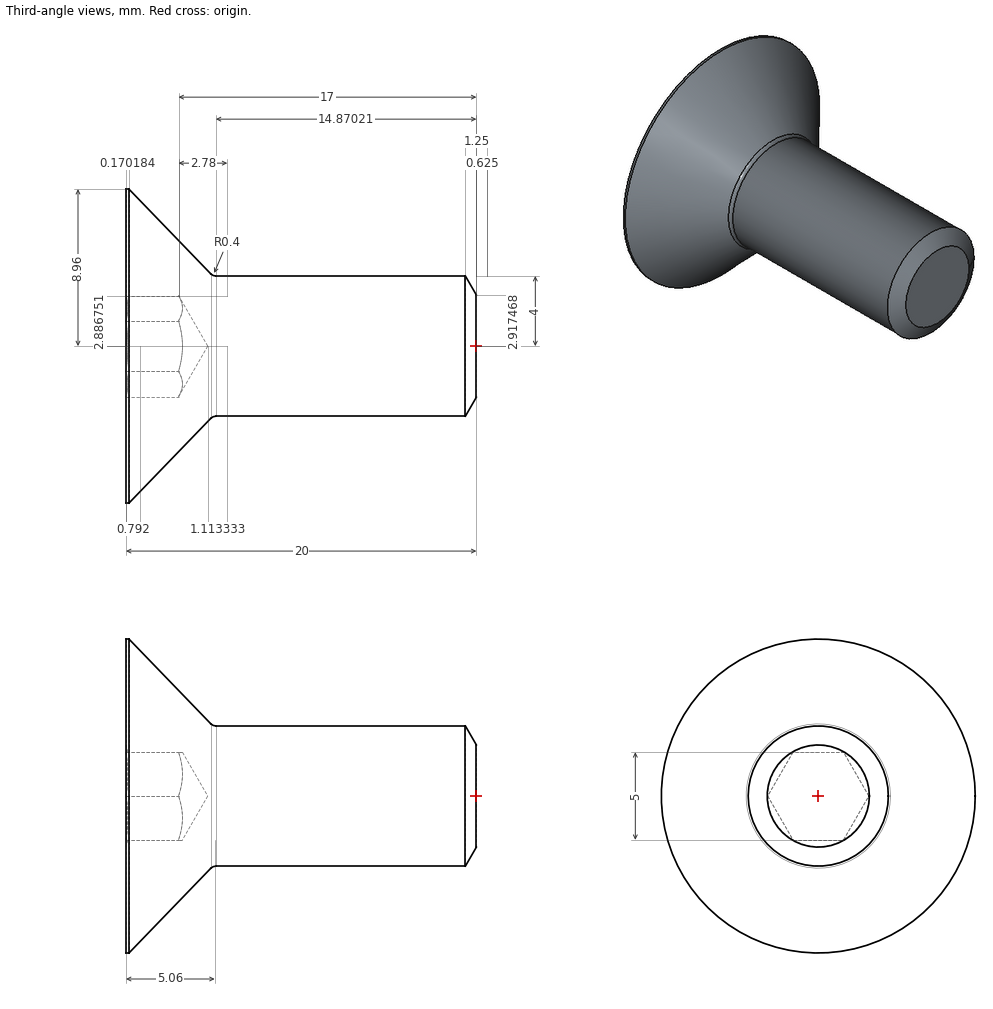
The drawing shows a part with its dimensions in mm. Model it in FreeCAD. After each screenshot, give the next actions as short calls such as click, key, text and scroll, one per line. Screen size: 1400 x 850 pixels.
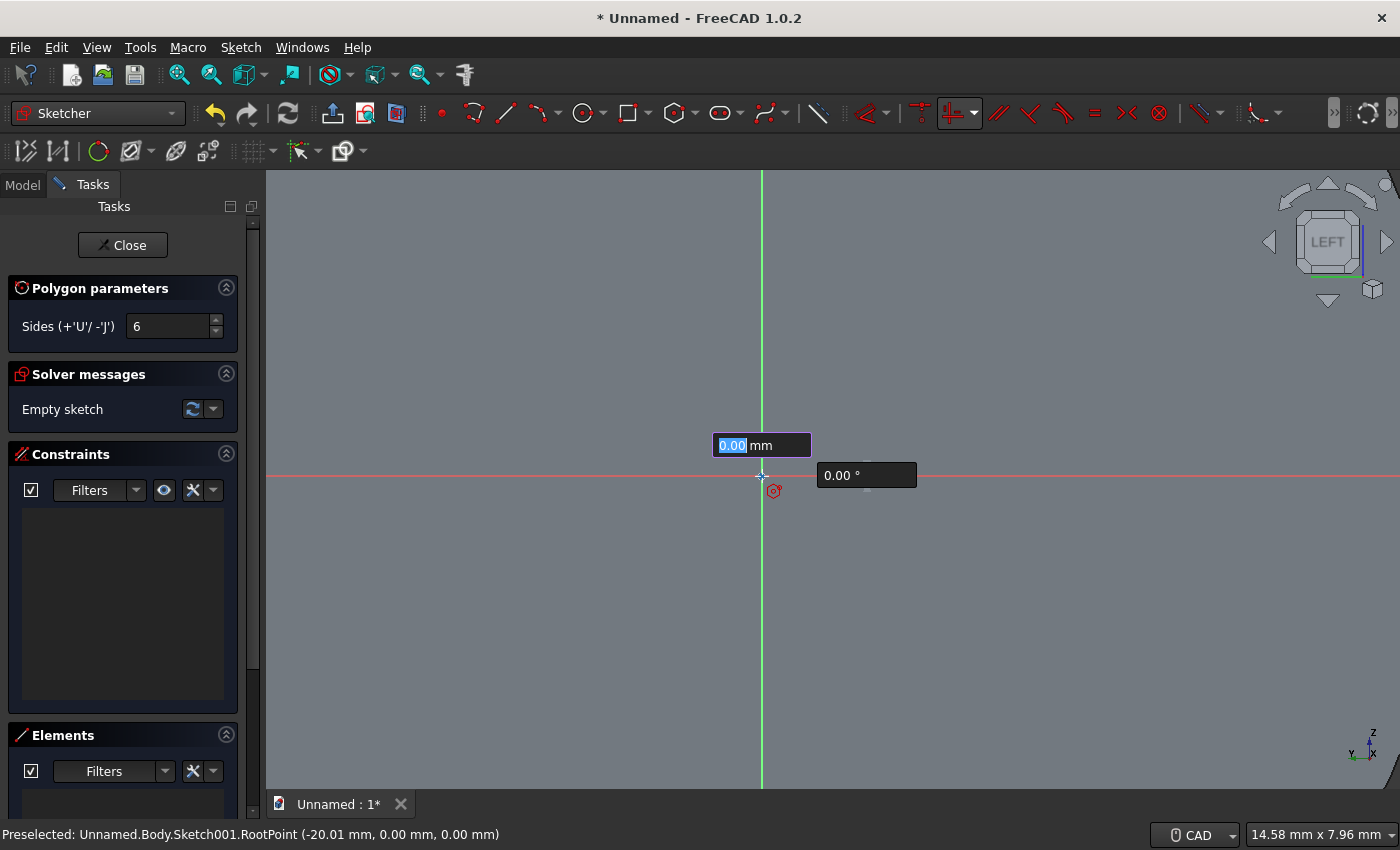
click(537, 476)
right_click(537, 476)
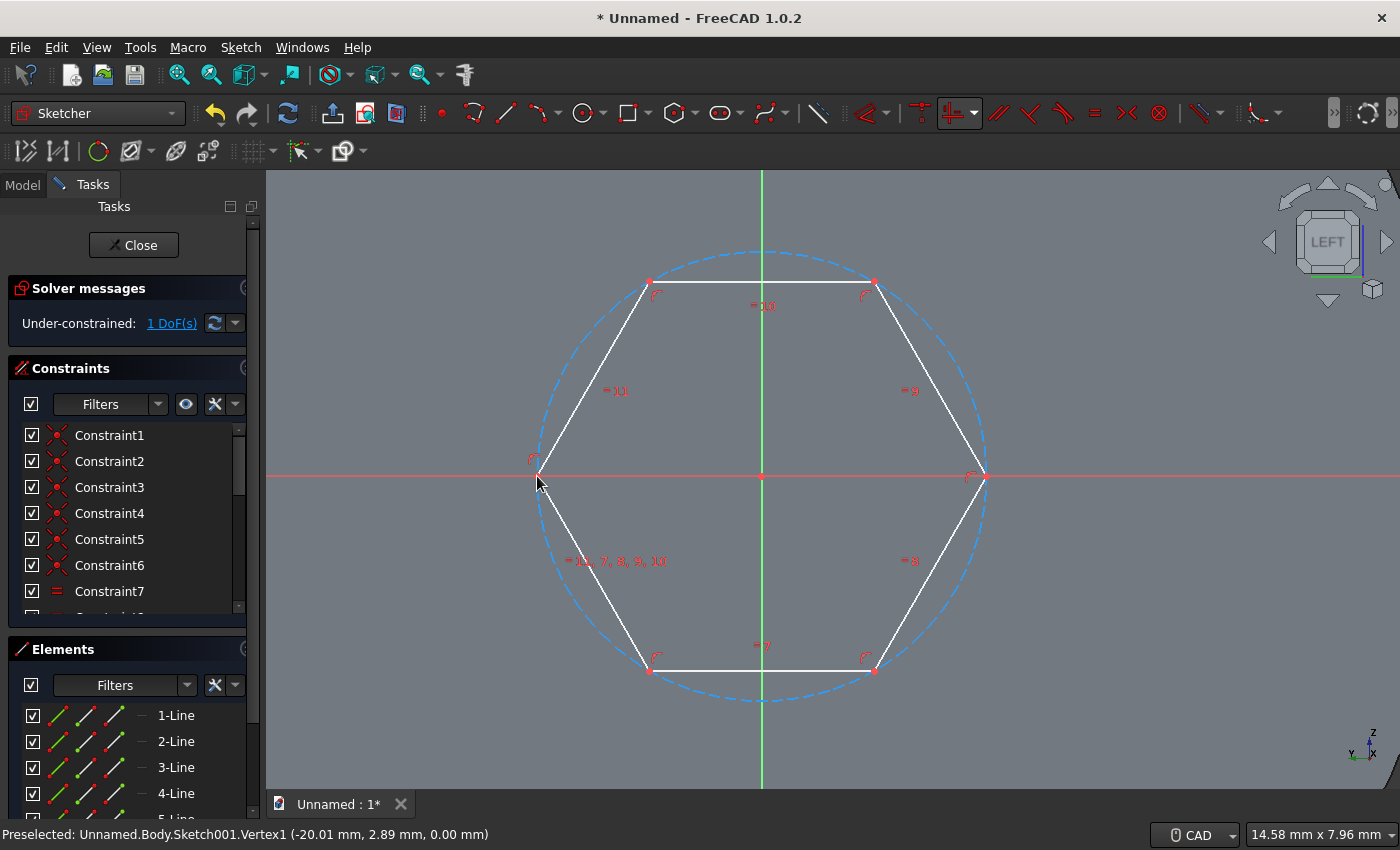
click(866, 114)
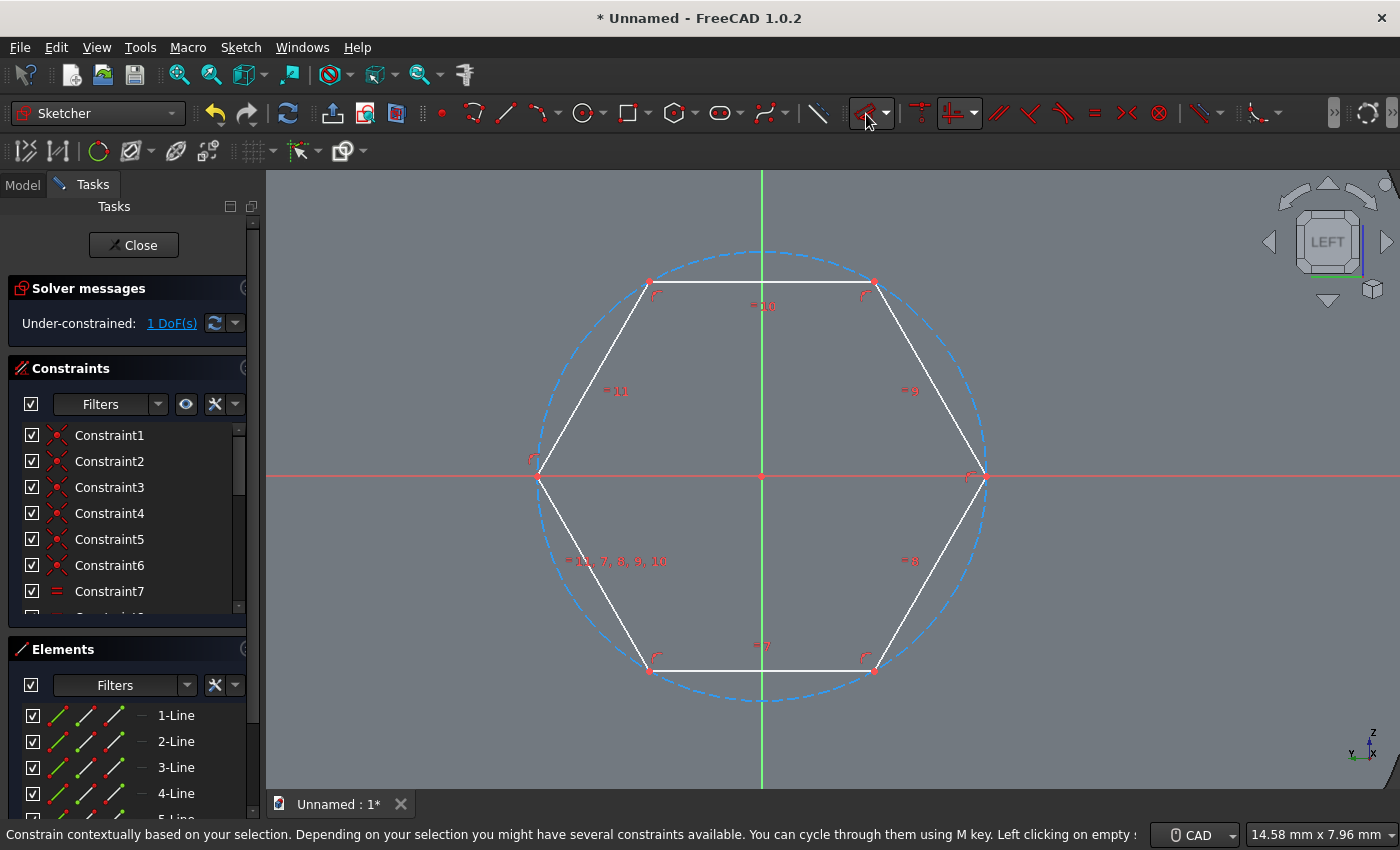
click(649, 671)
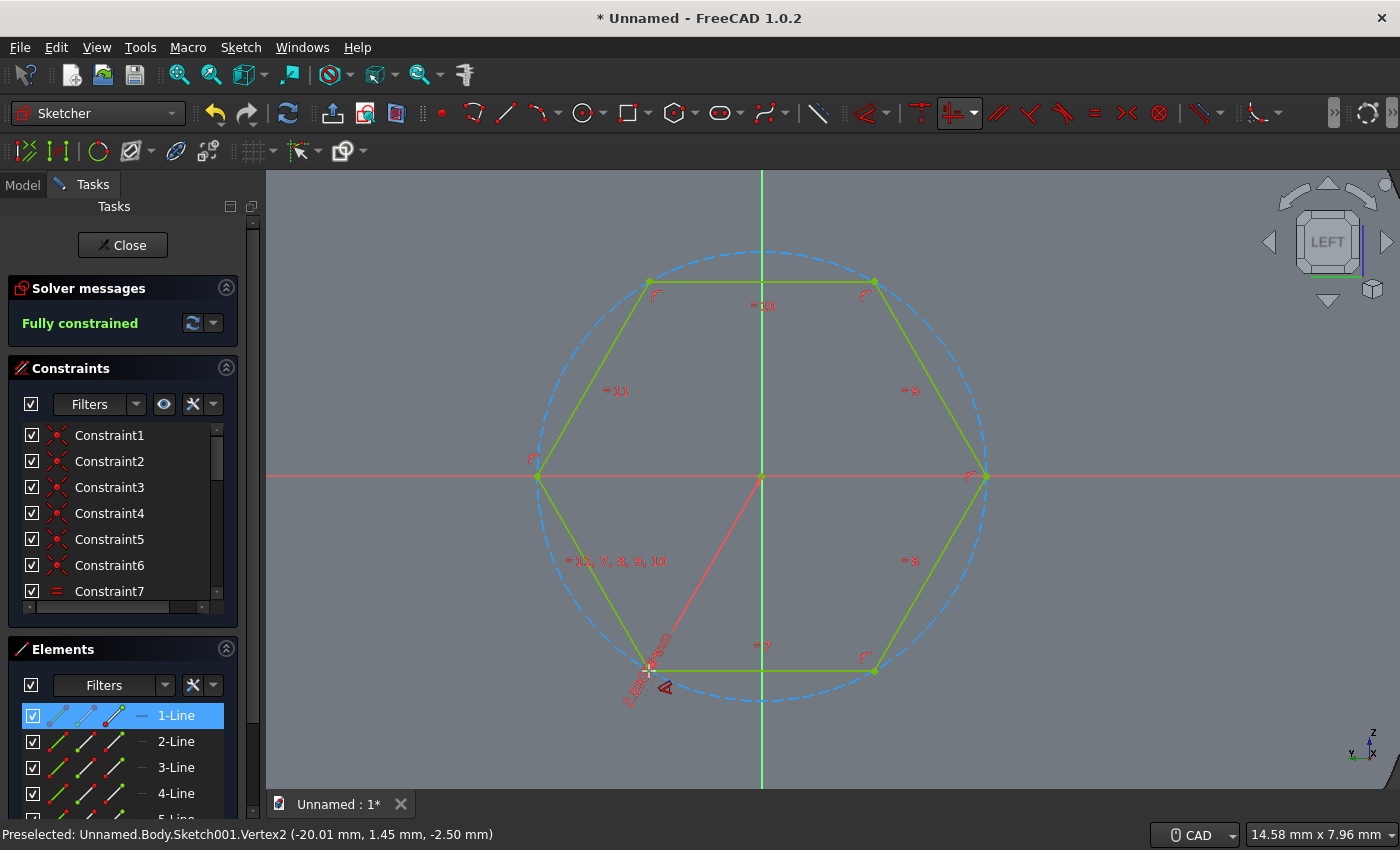
click(874, 282)
click(908, 387)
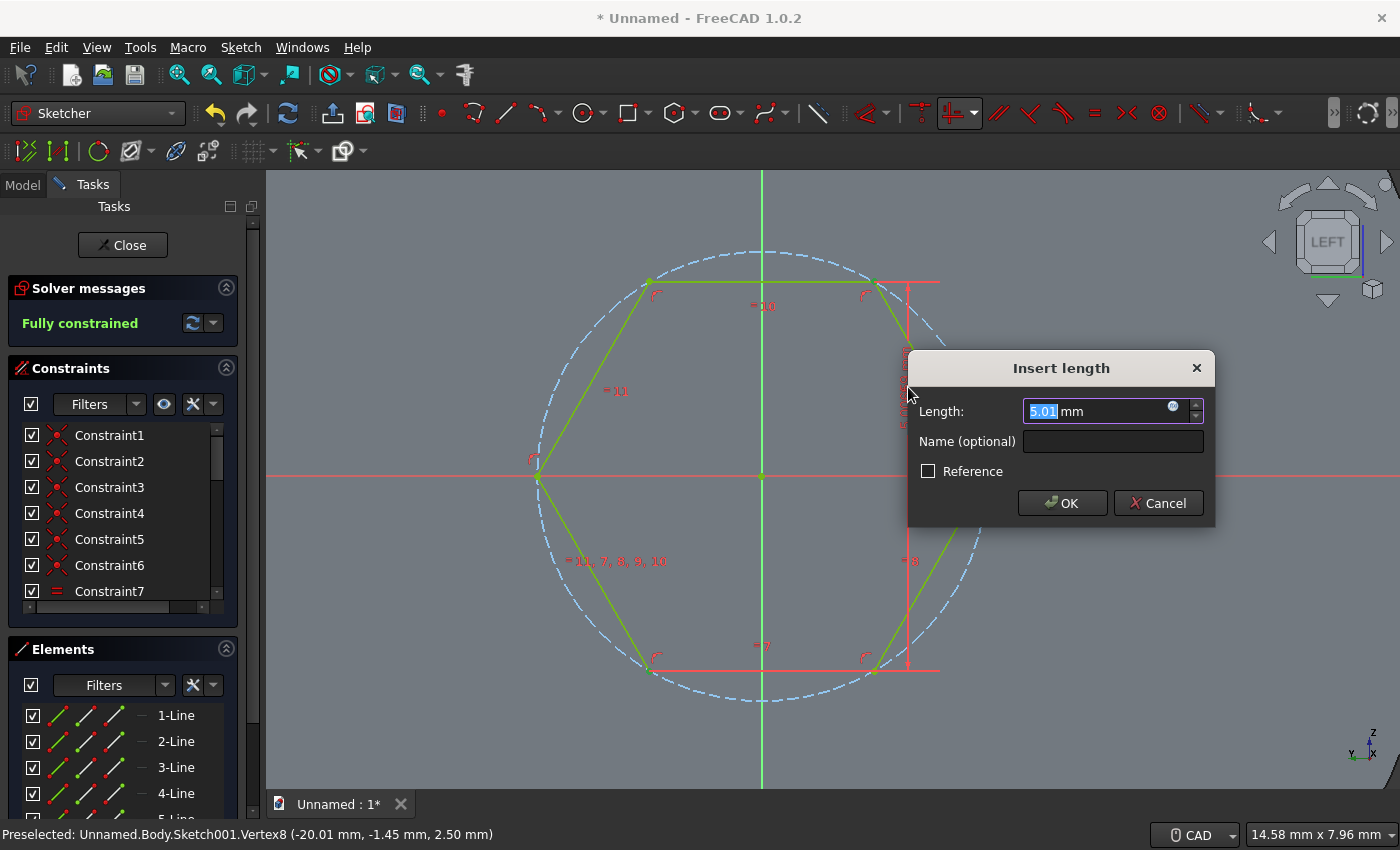
text(5)
key(Return)
key(Escape)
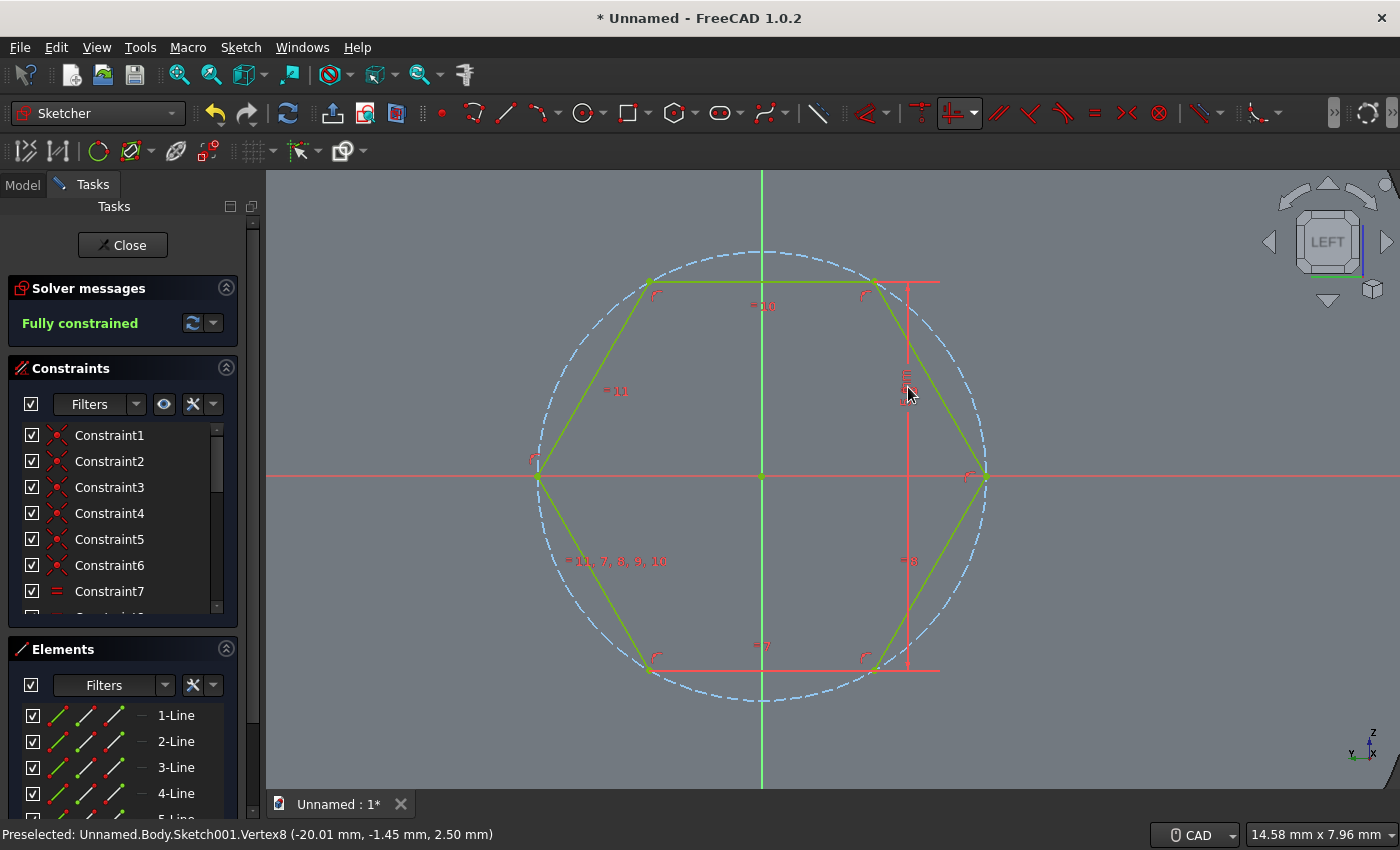
click(123, 245)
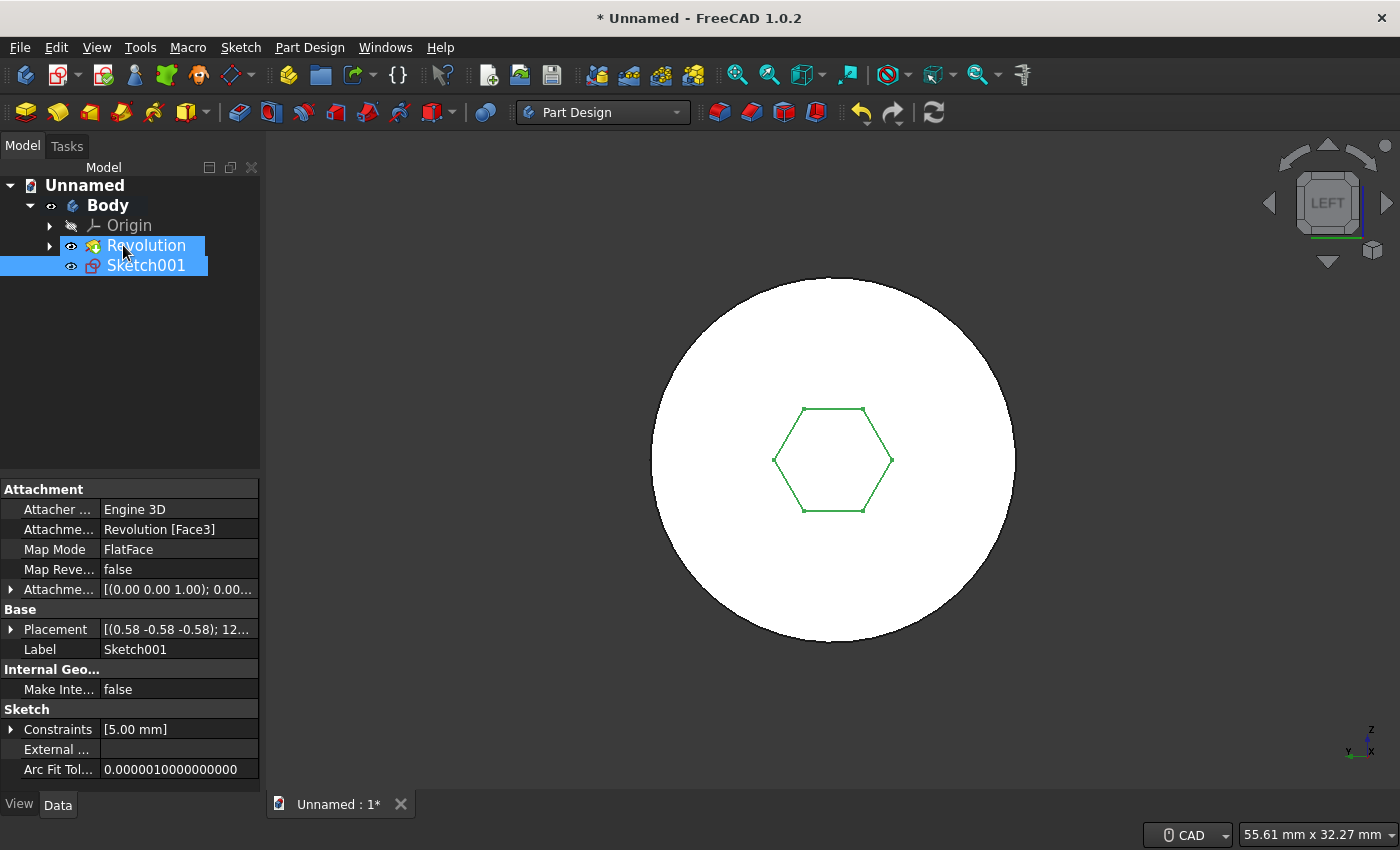
click(240, 112)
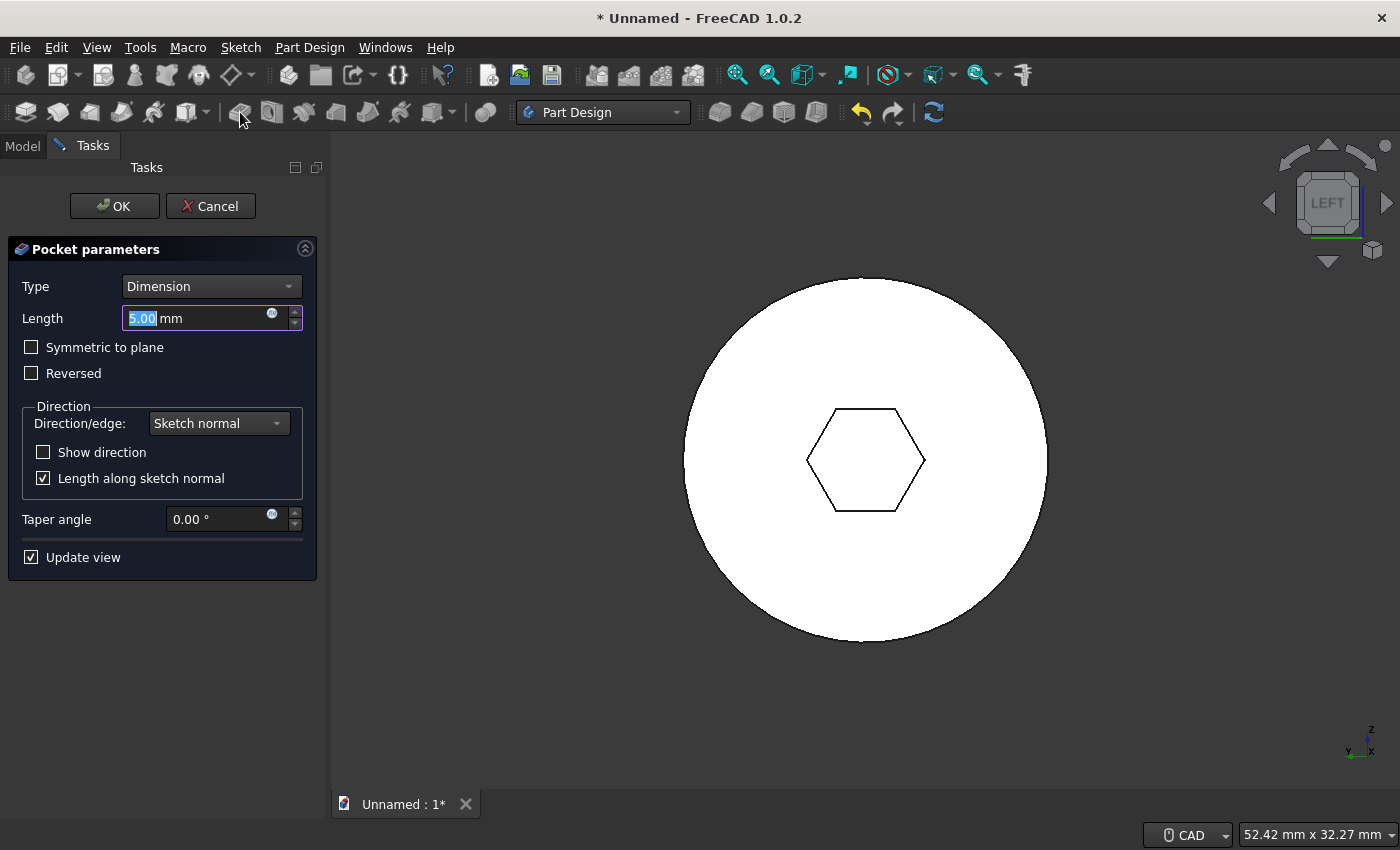
text(5.06)
key(Tab)